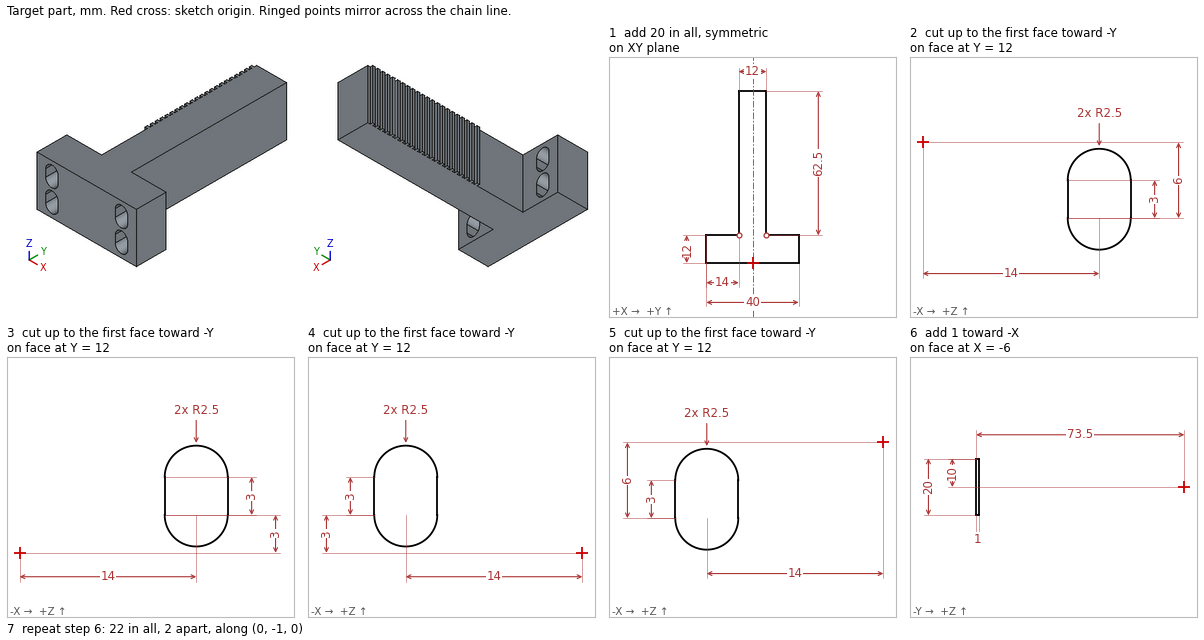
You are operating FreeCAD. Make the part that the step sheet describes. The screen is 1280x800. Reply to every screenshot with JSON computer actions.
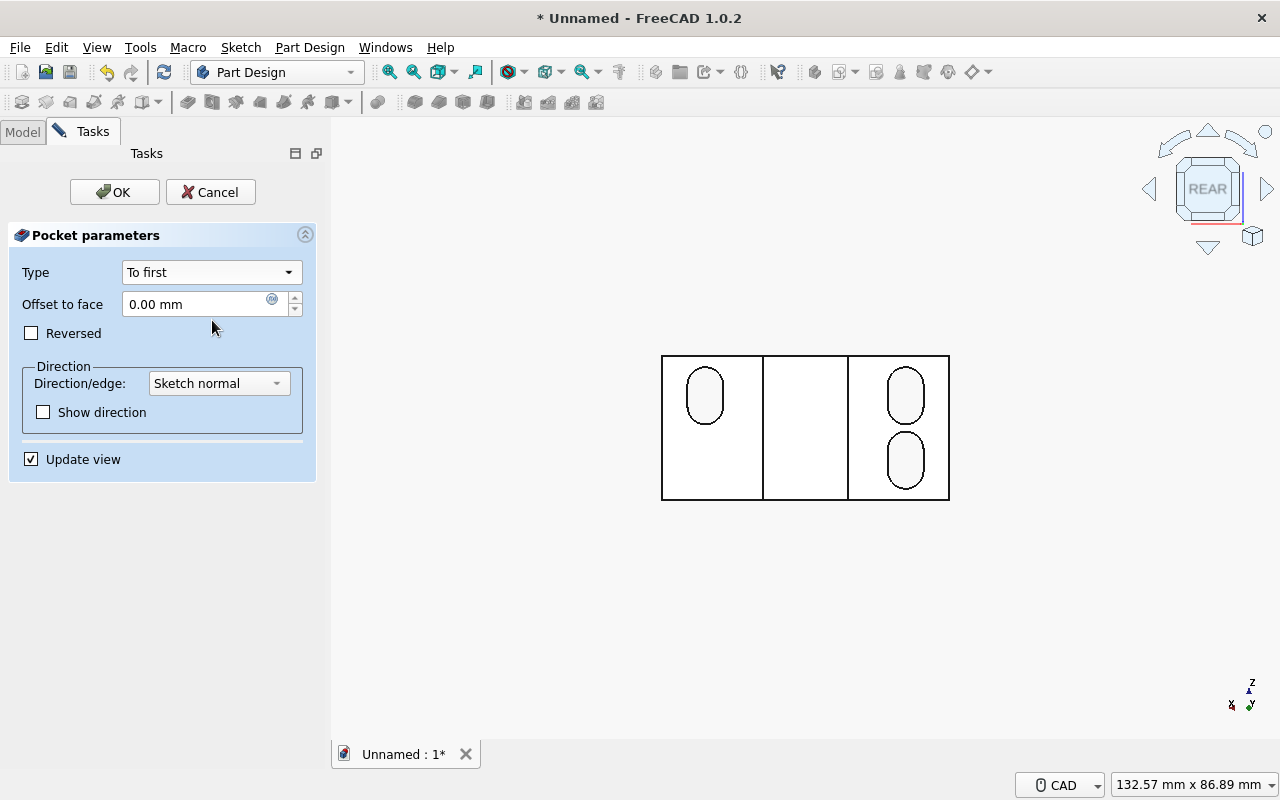
{"action": "left_click", "coordinate": [115, 192]}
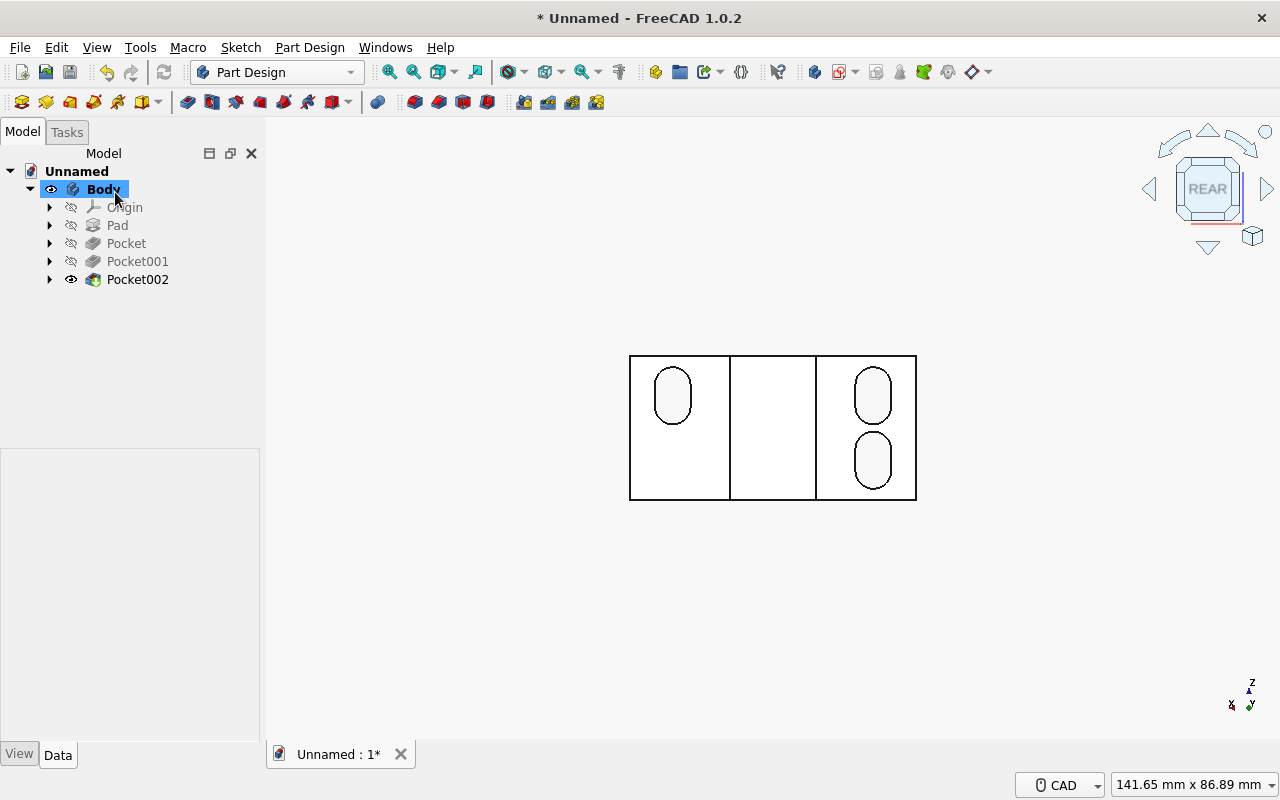
{"action": "key", "text": "v f"}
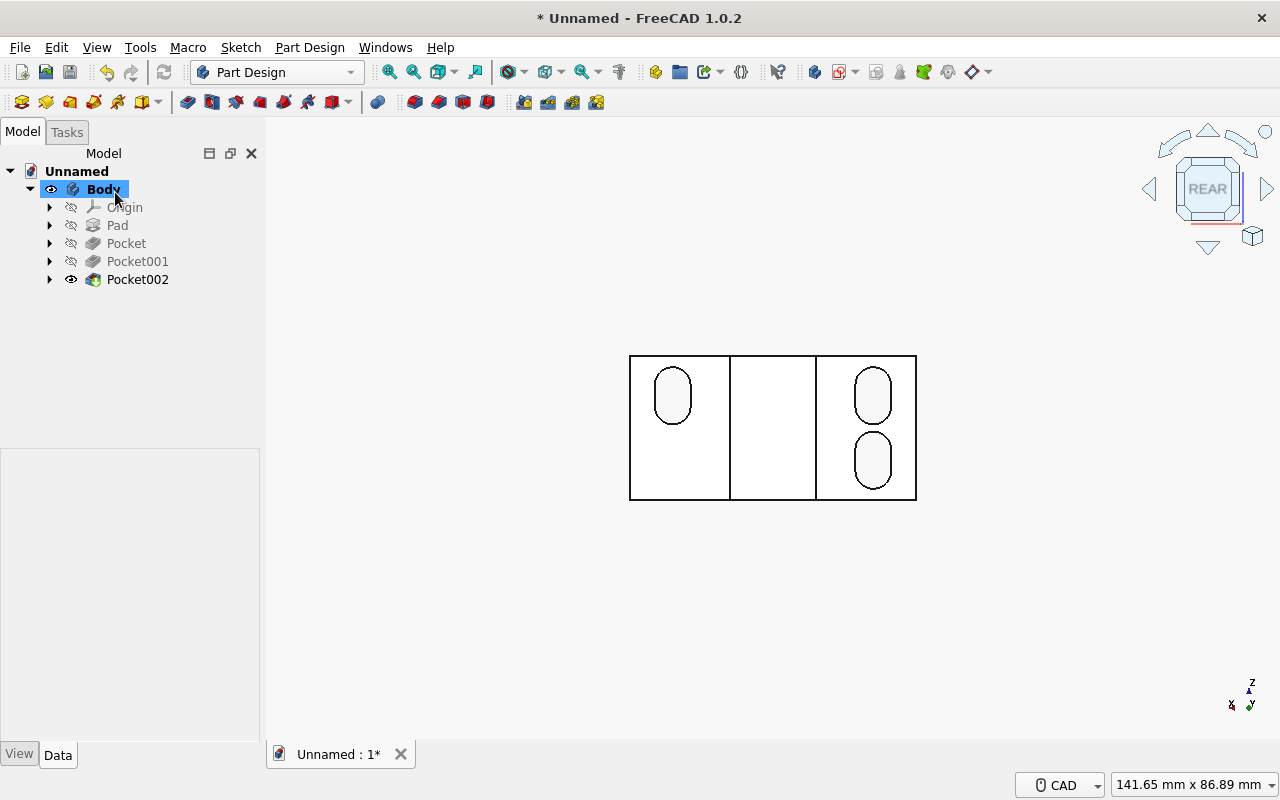
{"action": "left_click", "coordinate": [666, 468]}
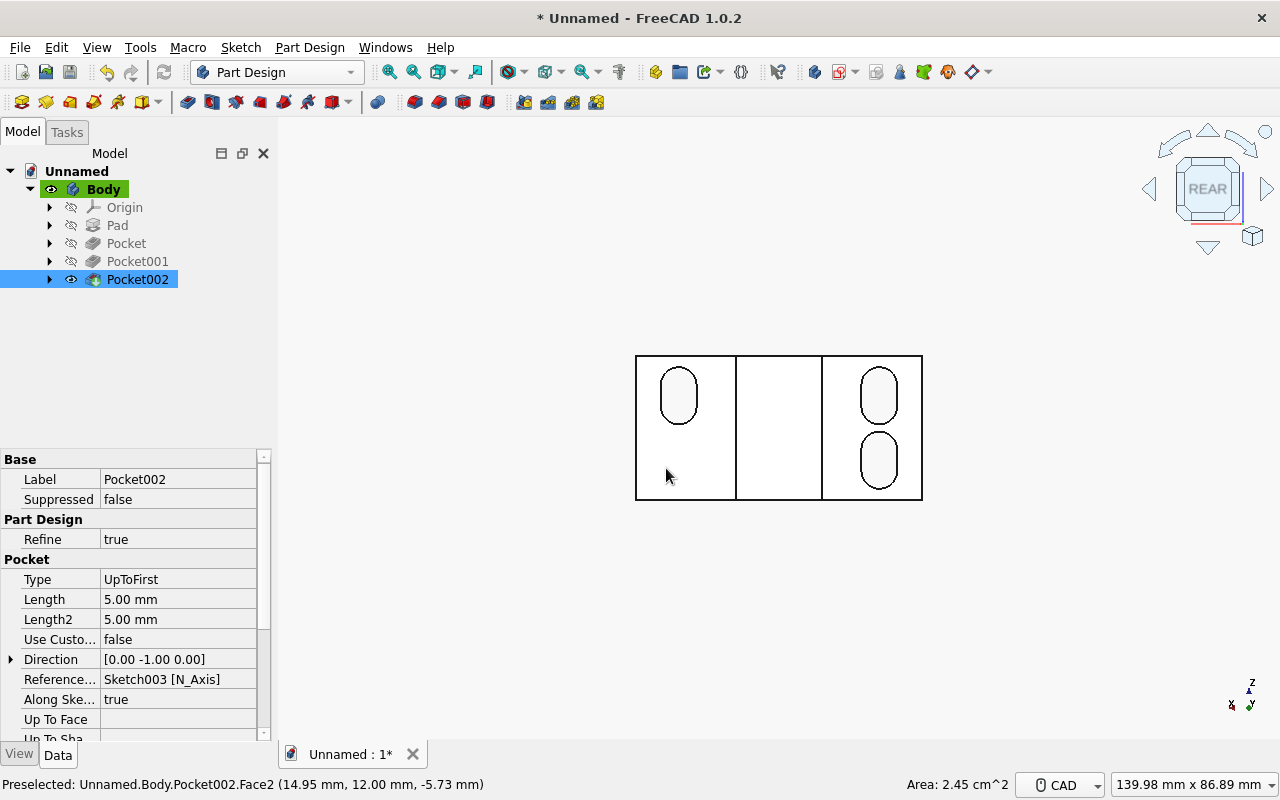
{"action": "left_click", "coordinate": [840, 72]}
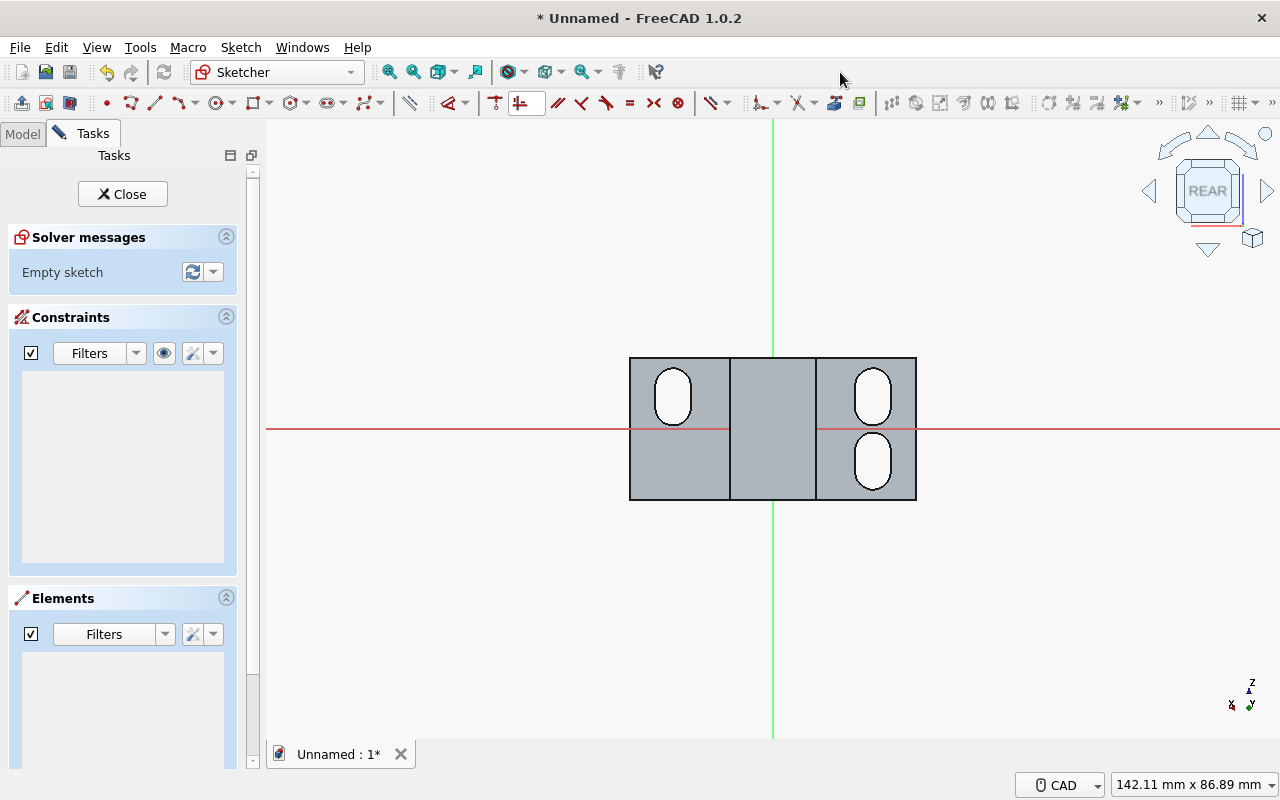
{"action": "key", "text": "q s"}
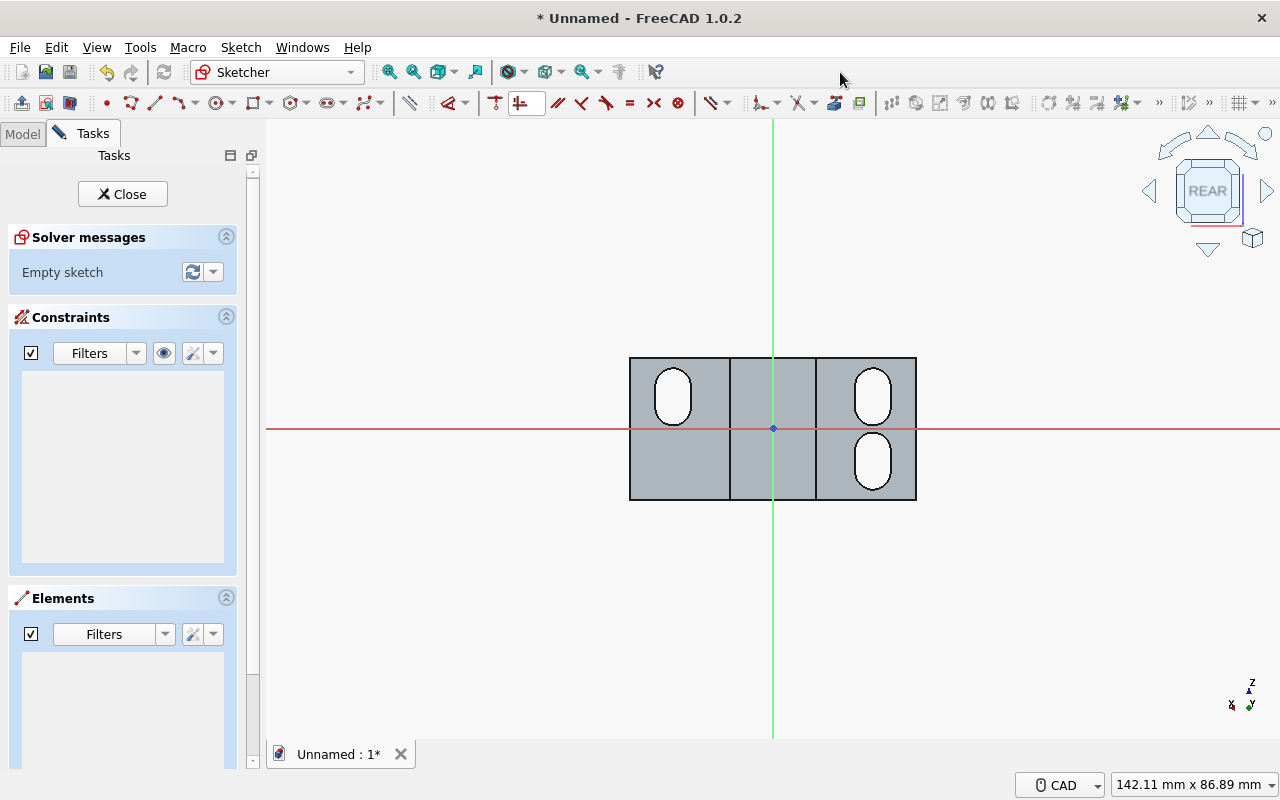
{"action": "scroll", "coordinate": [717, 467], "scroll_direction": "up", "scroll_amount": 8}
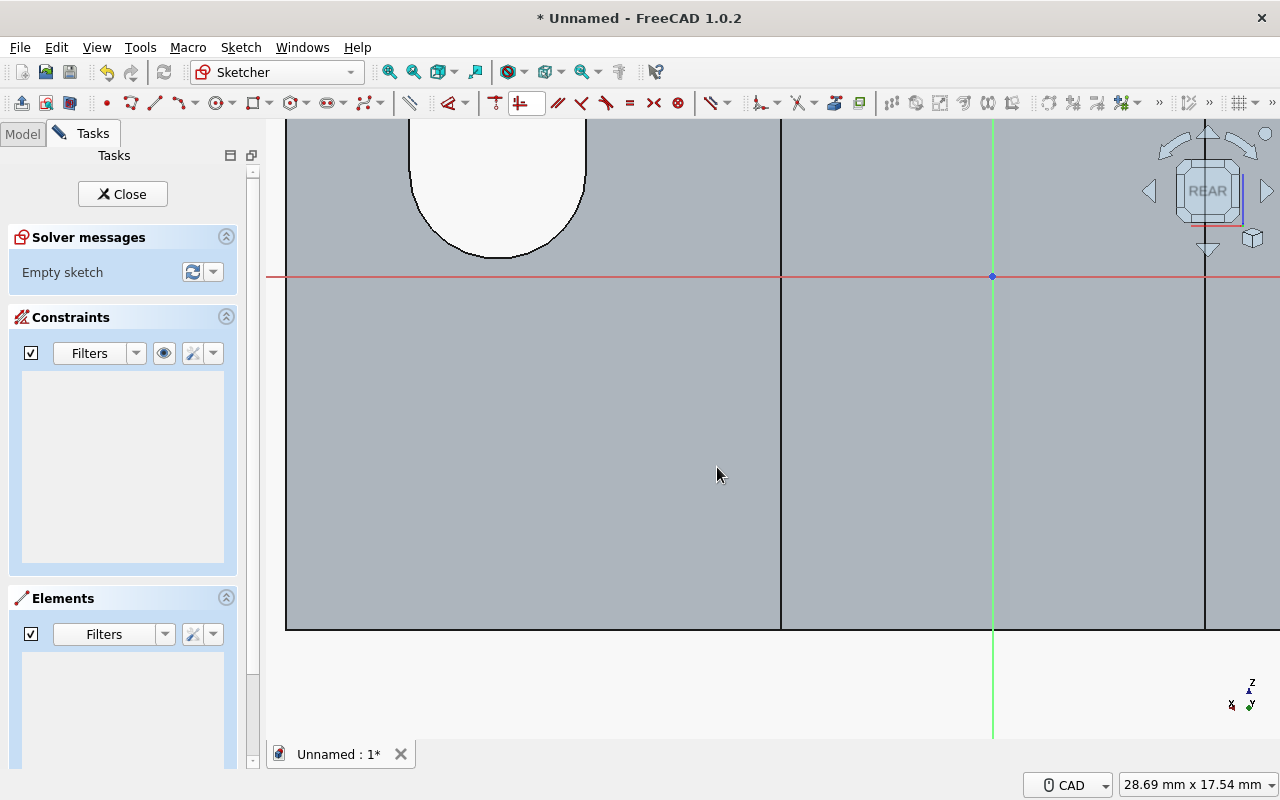
{"action": "left_click", "coordinate": [328, 104]}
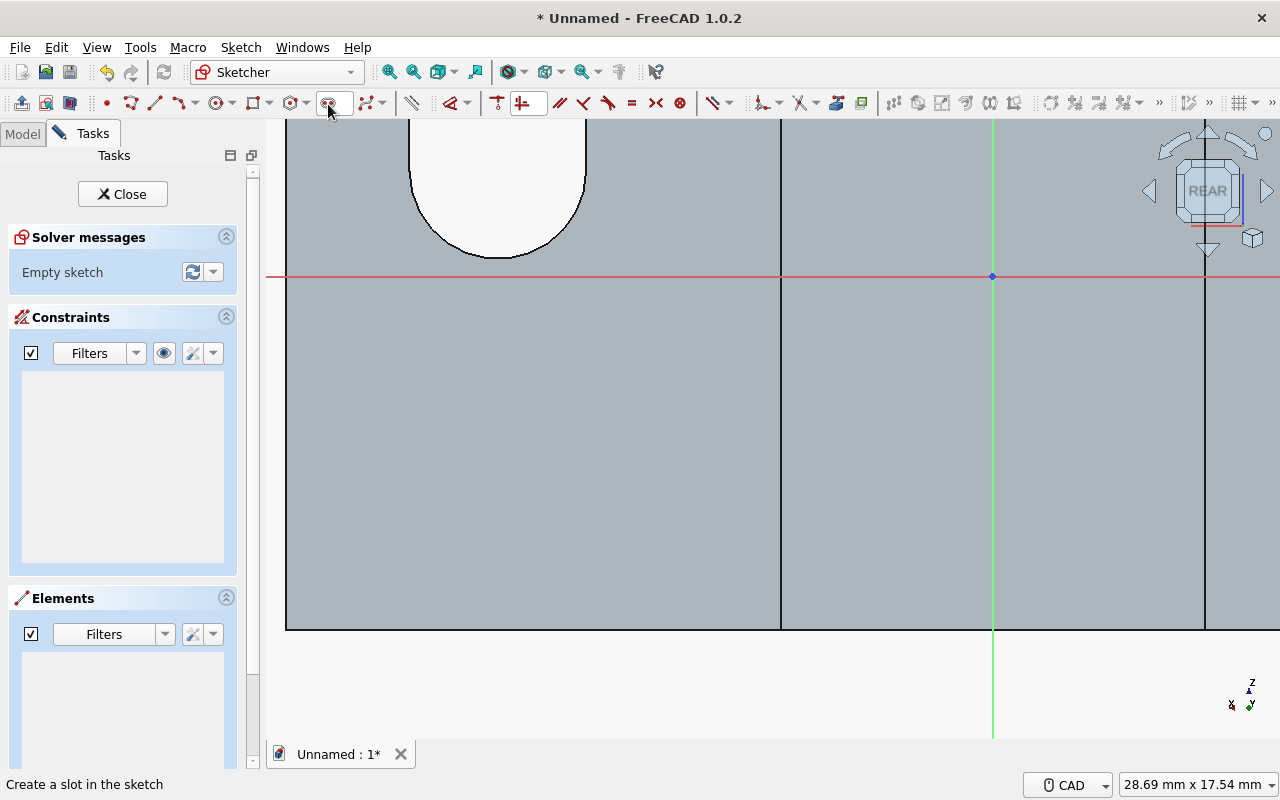
{"action": "left_click", "coordinate": [498, 489]}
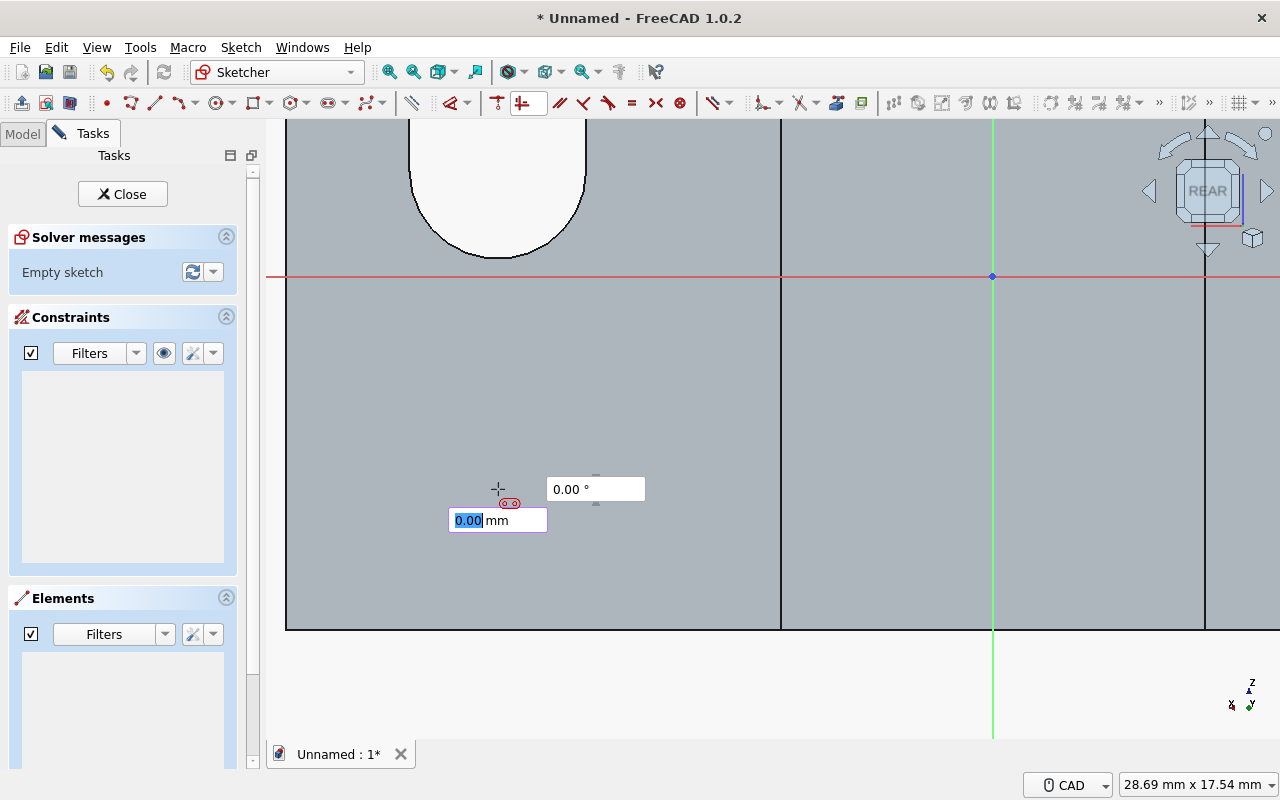
{"action": "left_click", "coordinate": [498, 383]}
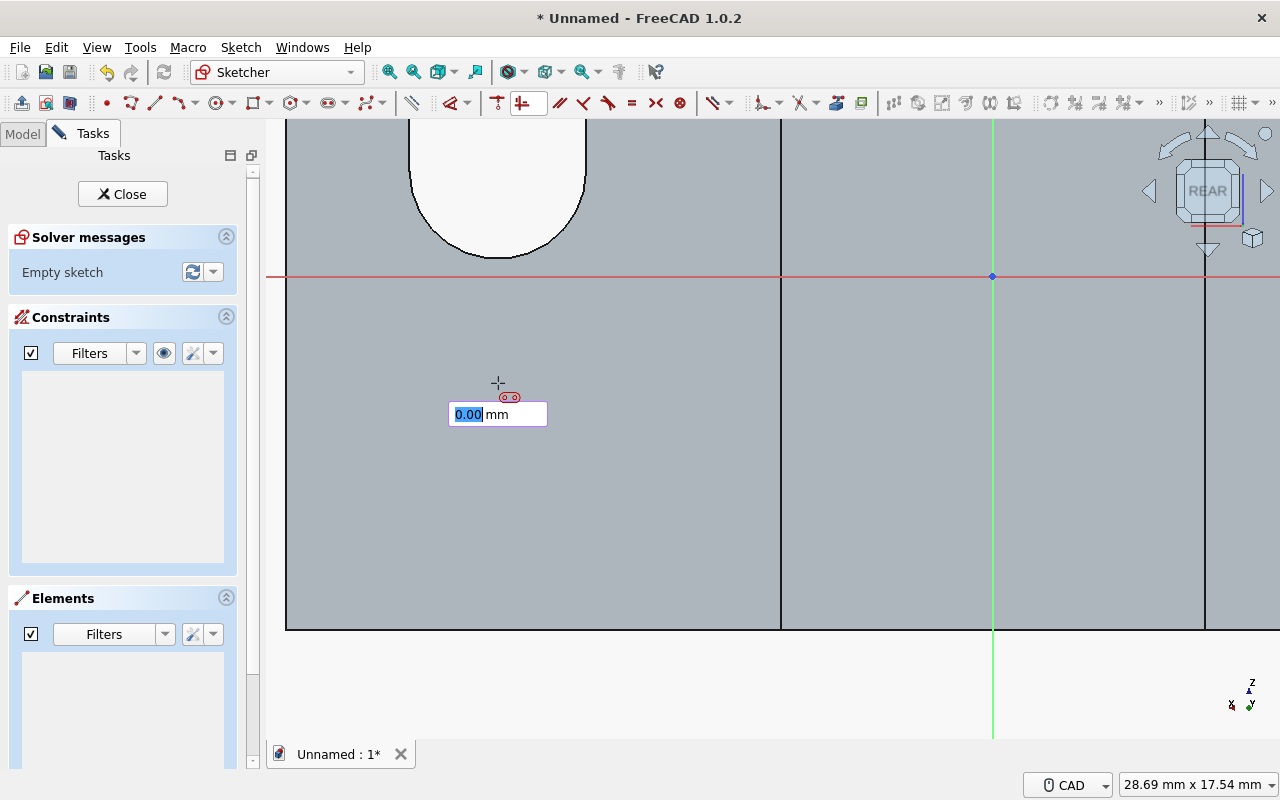
{"action": "left_click", "coordinate": [409, 436]}
{"action": "key", "text": "Escape"}